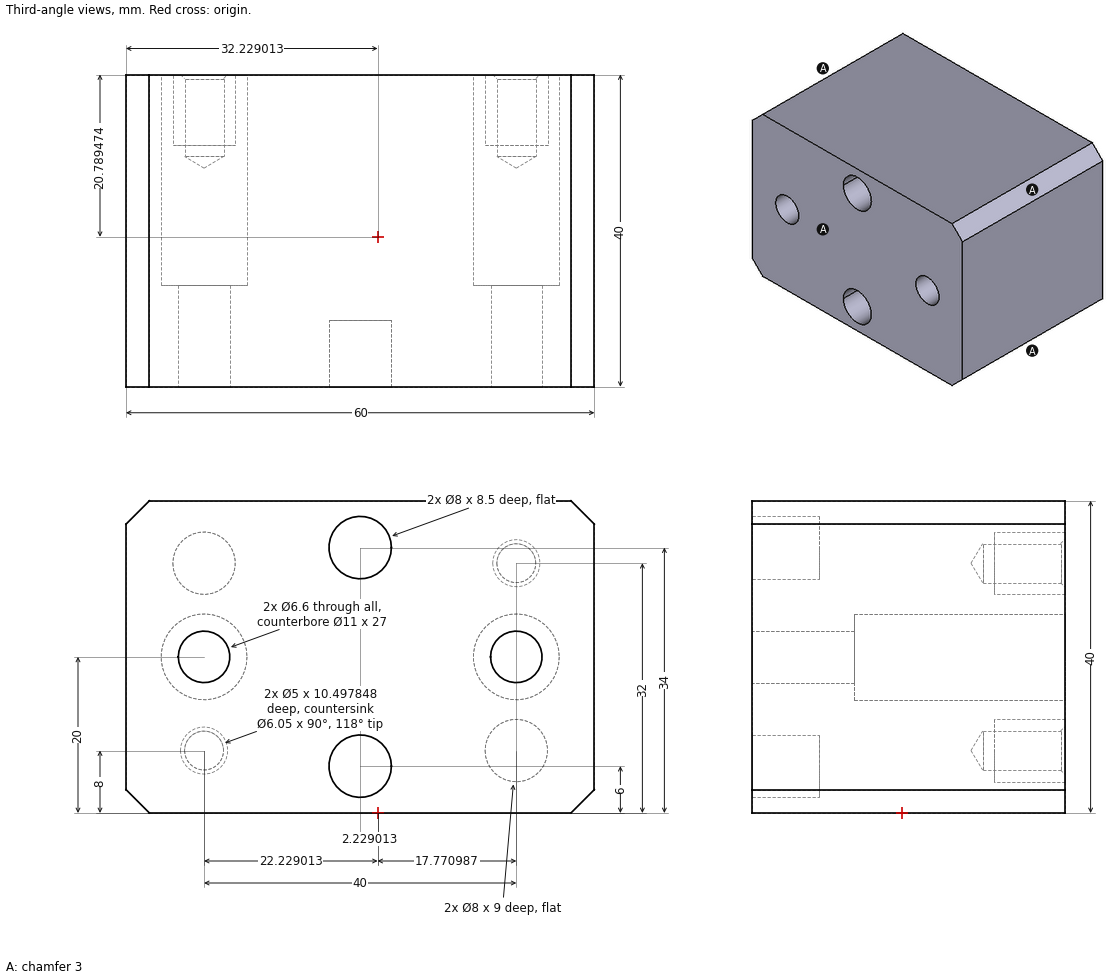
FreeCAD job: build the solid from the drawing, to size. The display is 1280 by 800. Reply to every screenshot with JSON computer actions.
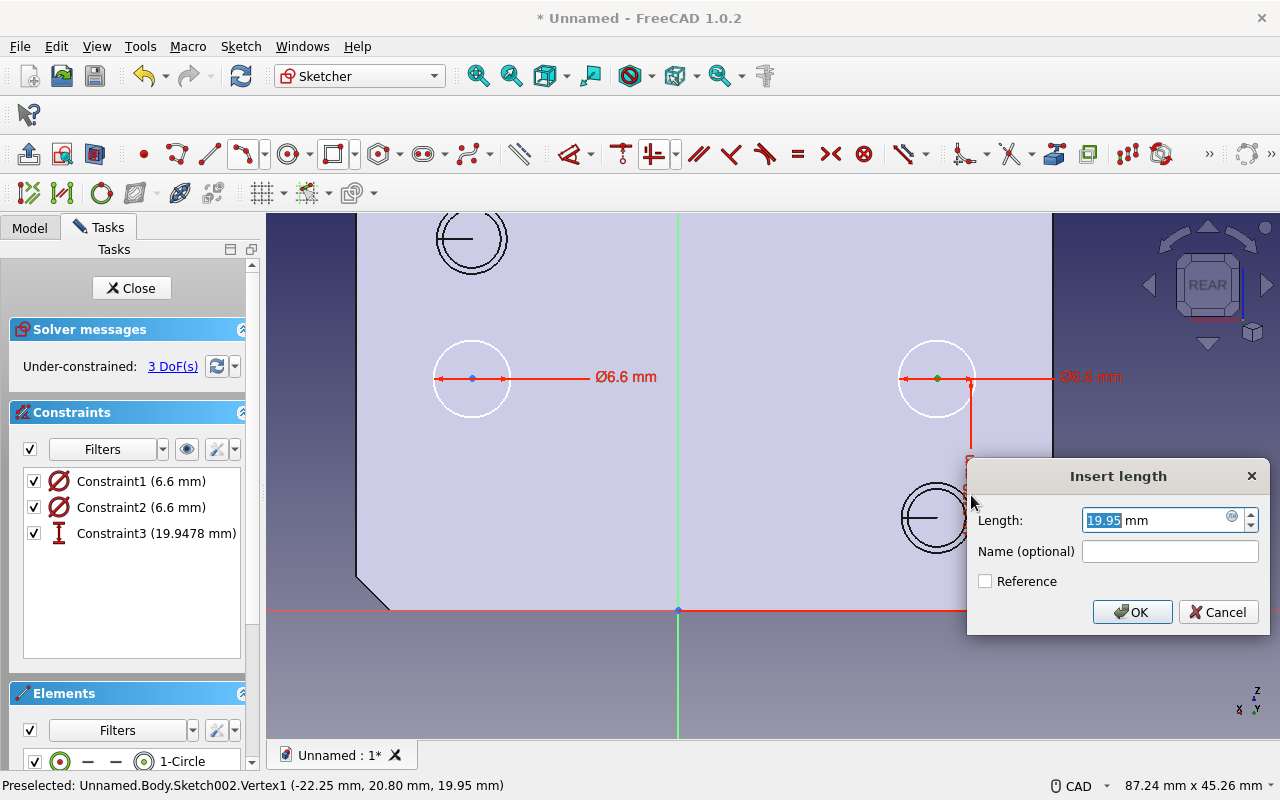
{"action": "type", "text": "20"}
{"action": "key", "text": "Return"}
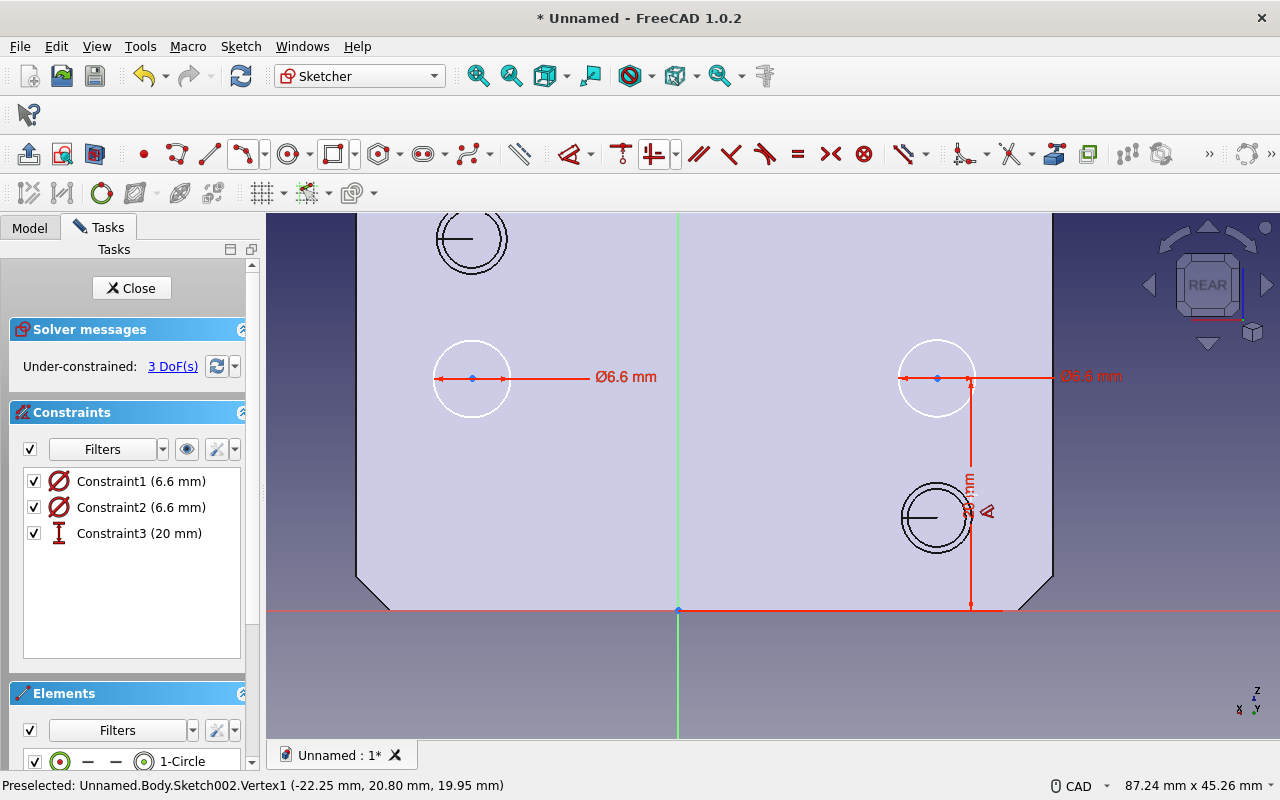
{"action": "left_click", "coordinate": [472, 379]}
{"action": "left_click", "coordinate": [438, 495]}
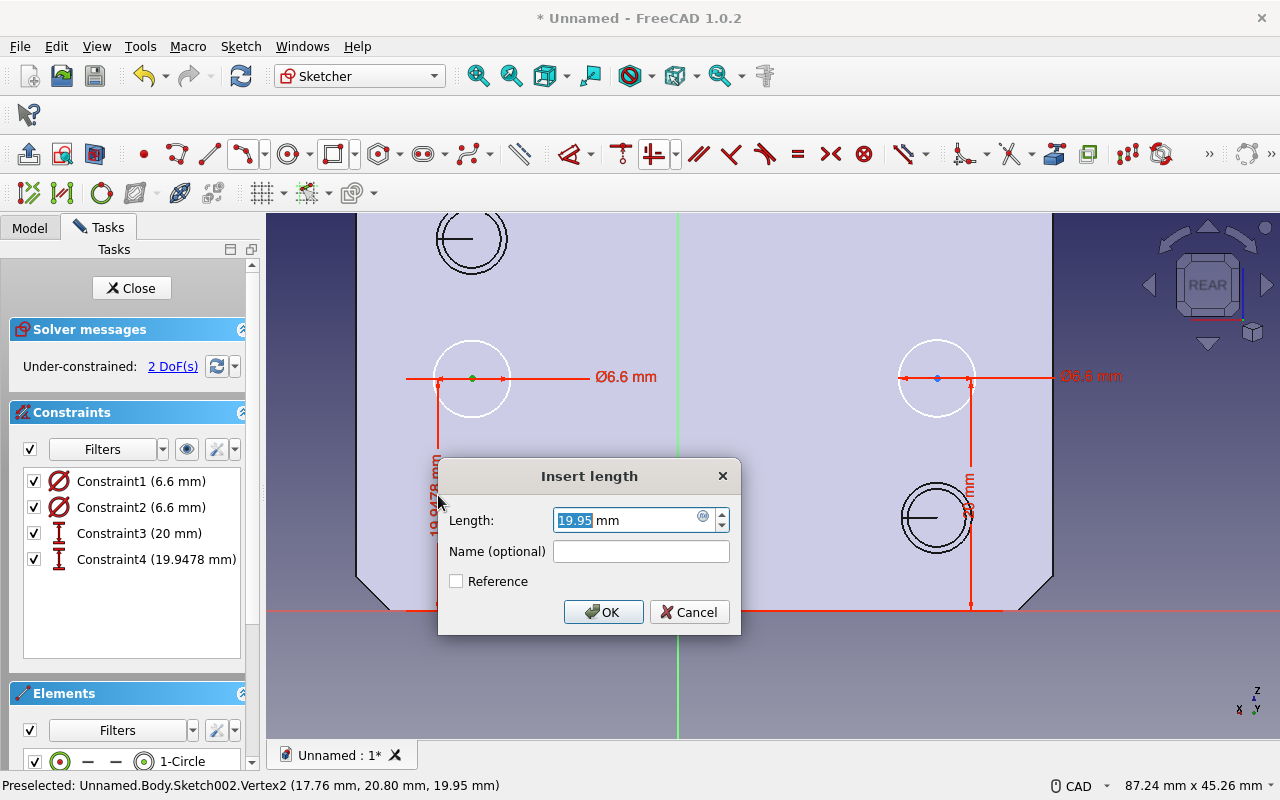
{"action": "type", "text": "20"}
{"action": "key", "text": "Return"}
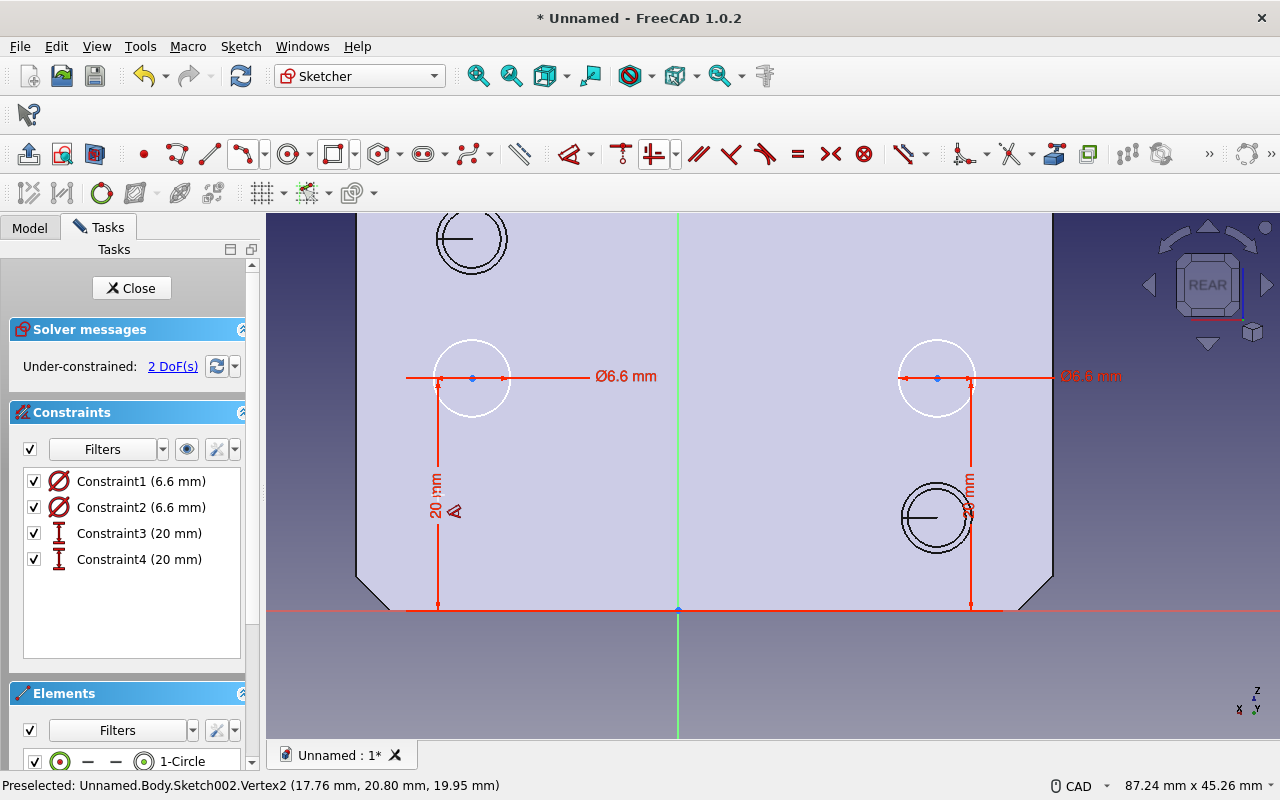
{"action": "left_click", "coordinate": [937, 378]}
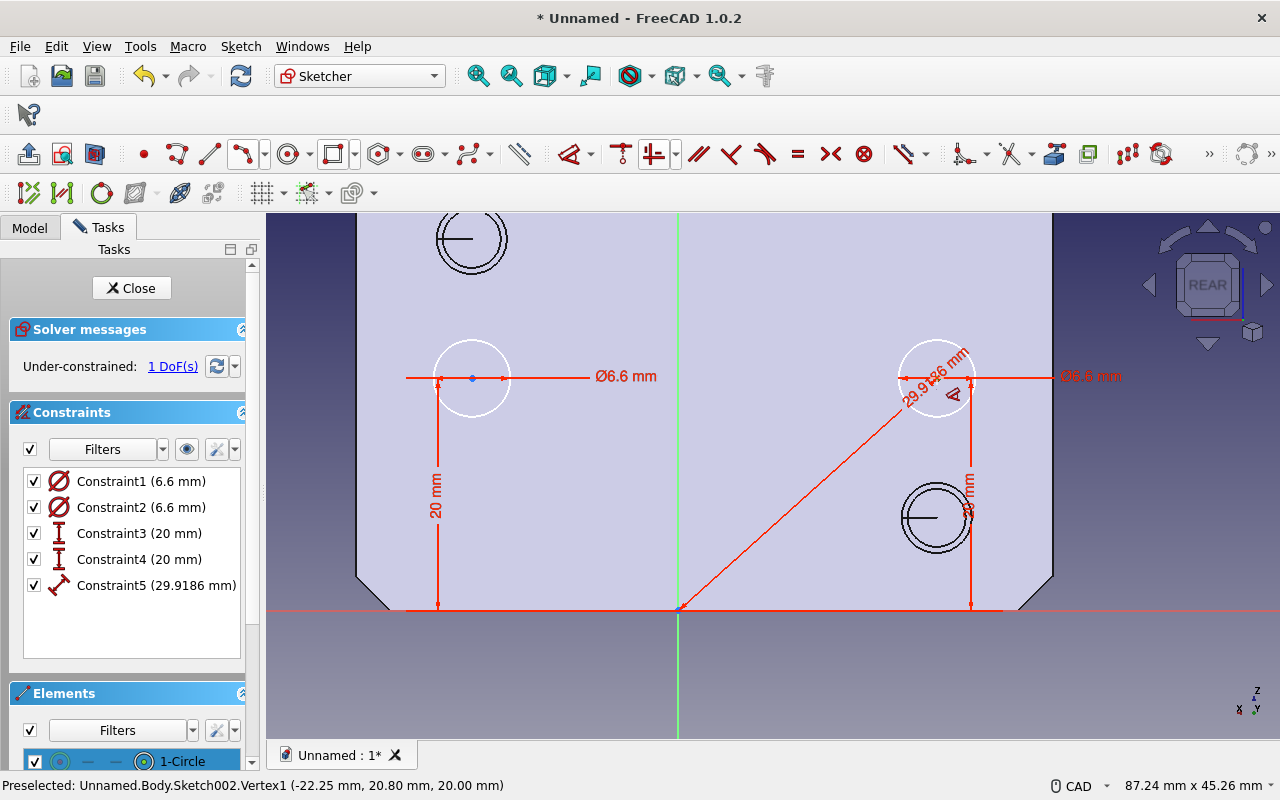
{"action": "left_click", "coordinate": [472, 378]}
{"action": "left_click", "coordinate": [705, 344]}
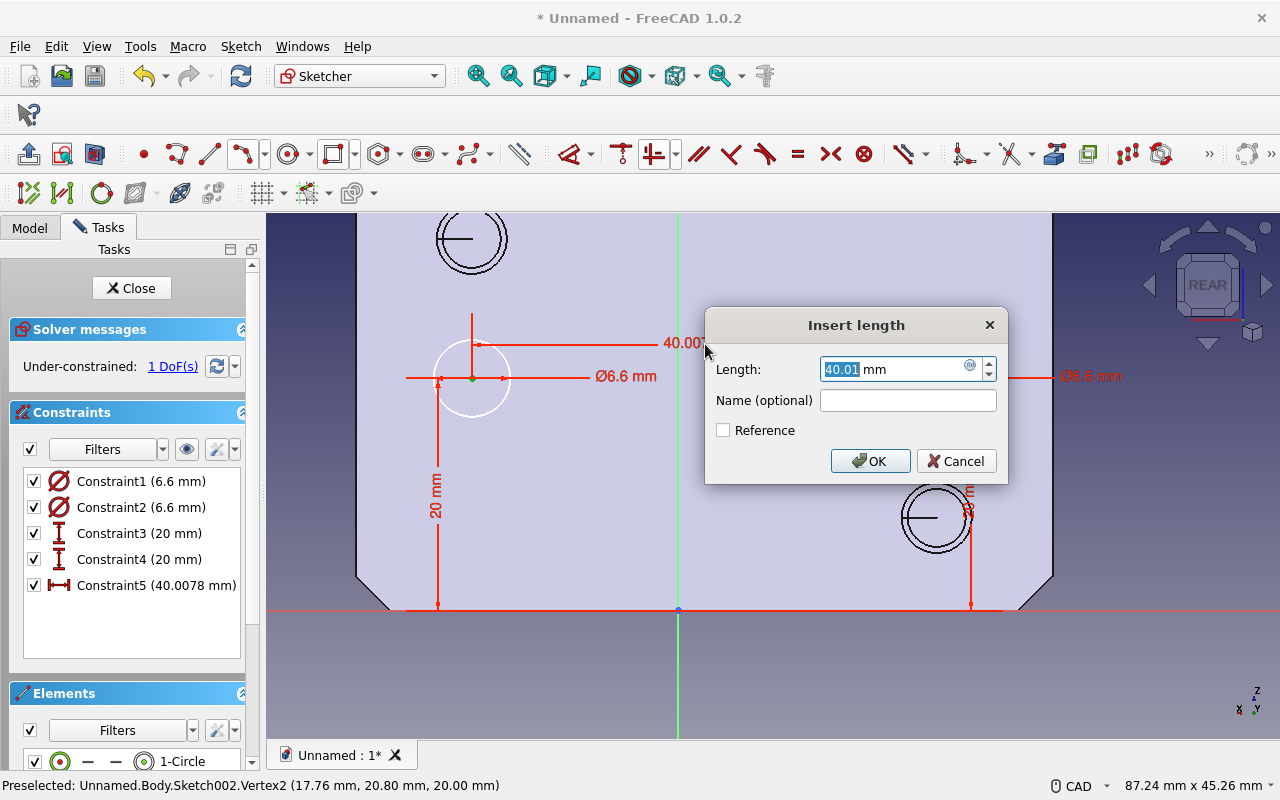
{"action": "type", "text": "40"}
{"action": "key", "text": "Return"}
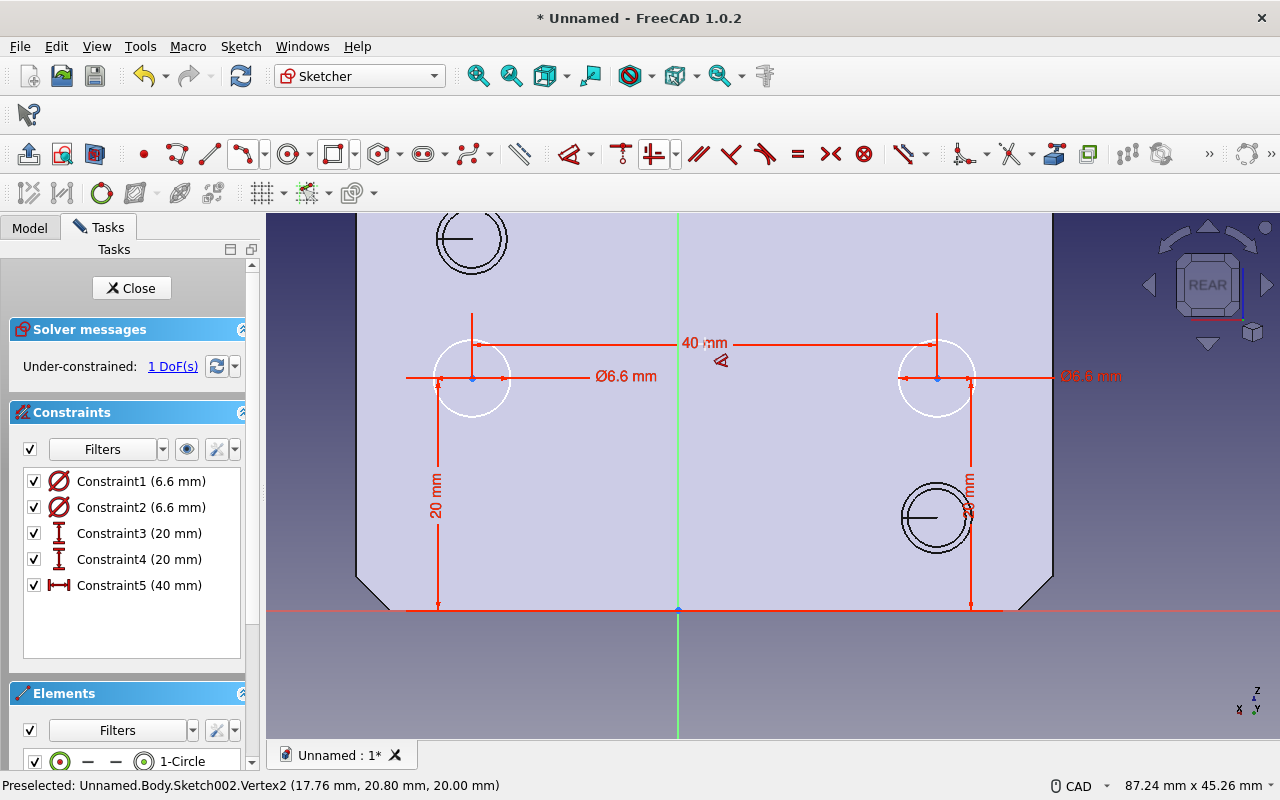
{"action": "left_click", "coordinate": [937, 378]}
{"action": "left_click", "coordinate": [808, 645]}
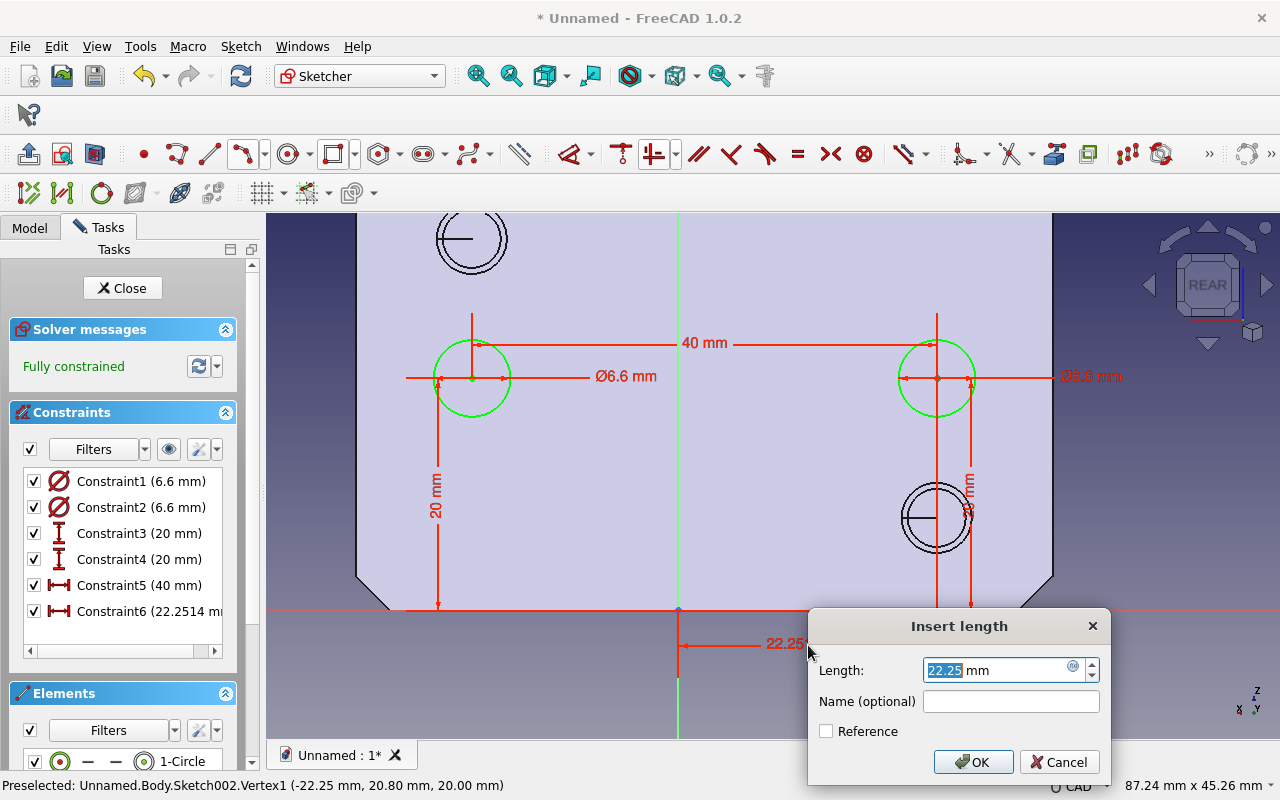
{"action": "type", "text": "22.229013"}
{"action": "key", "text": "Return"}
{"action": "key", "text": "Escape"}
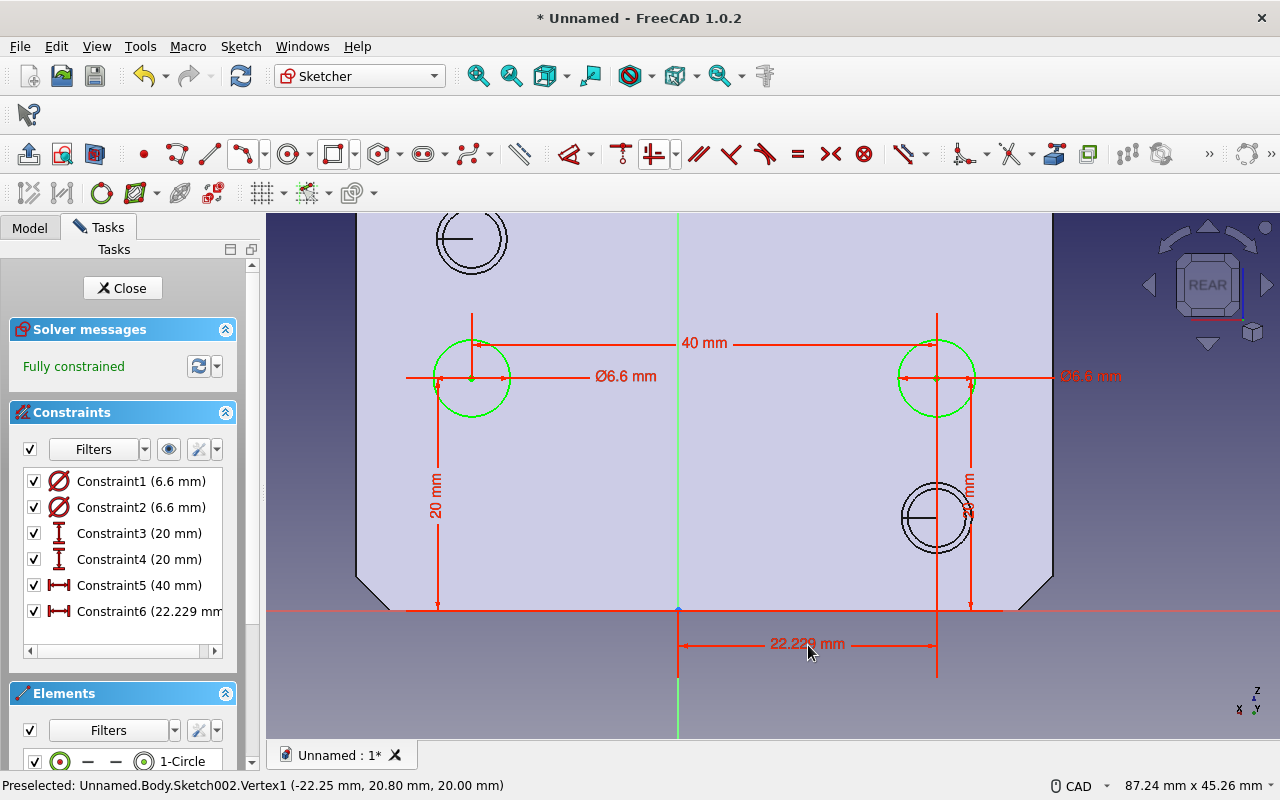
{"action": "left_click", "coordinate": [123, 288]}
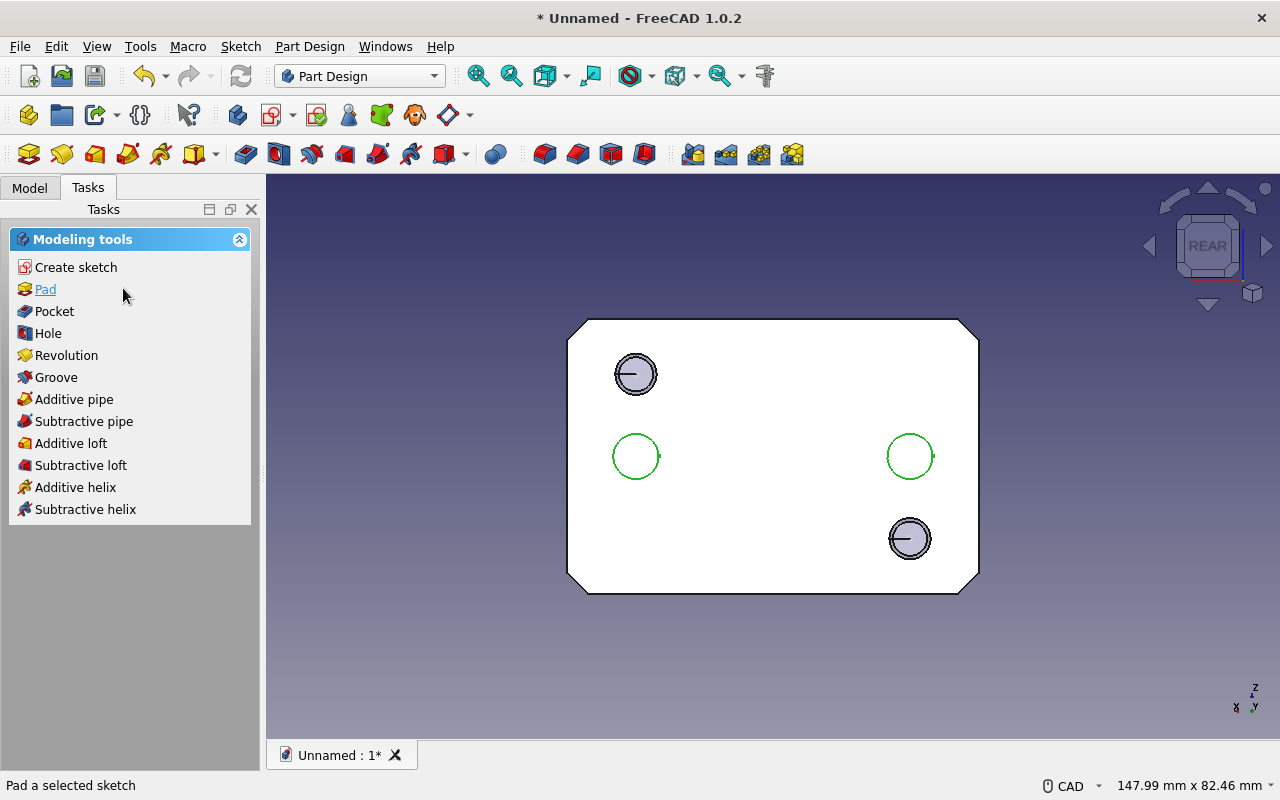
{"action": "left_click", "coordinate": [279, 154]}